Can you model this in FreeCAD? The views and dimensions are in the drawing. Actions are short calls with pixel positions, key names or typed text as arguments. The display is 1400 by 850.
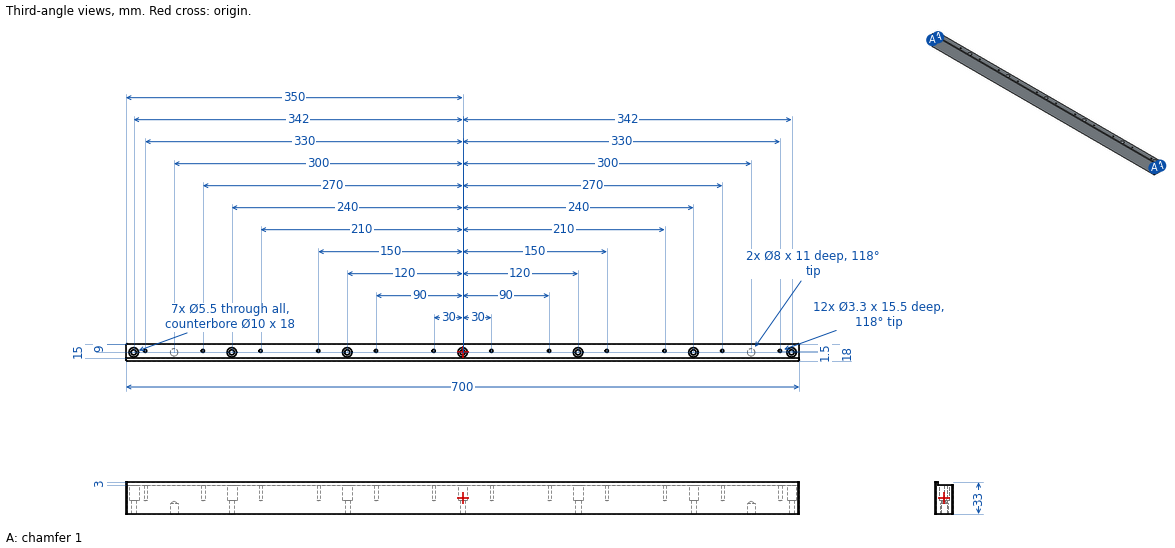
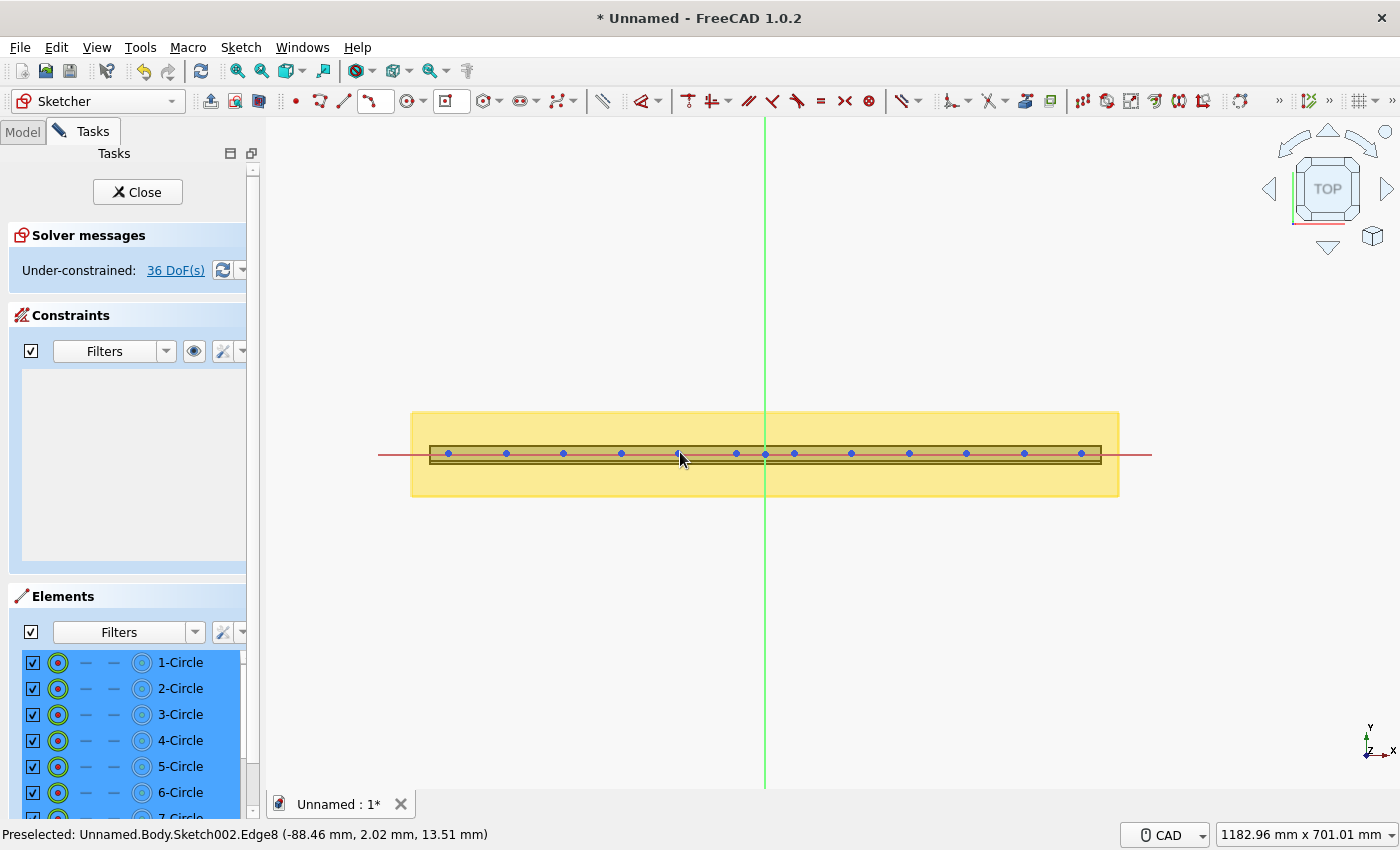
scroll(623, 452, up, 11)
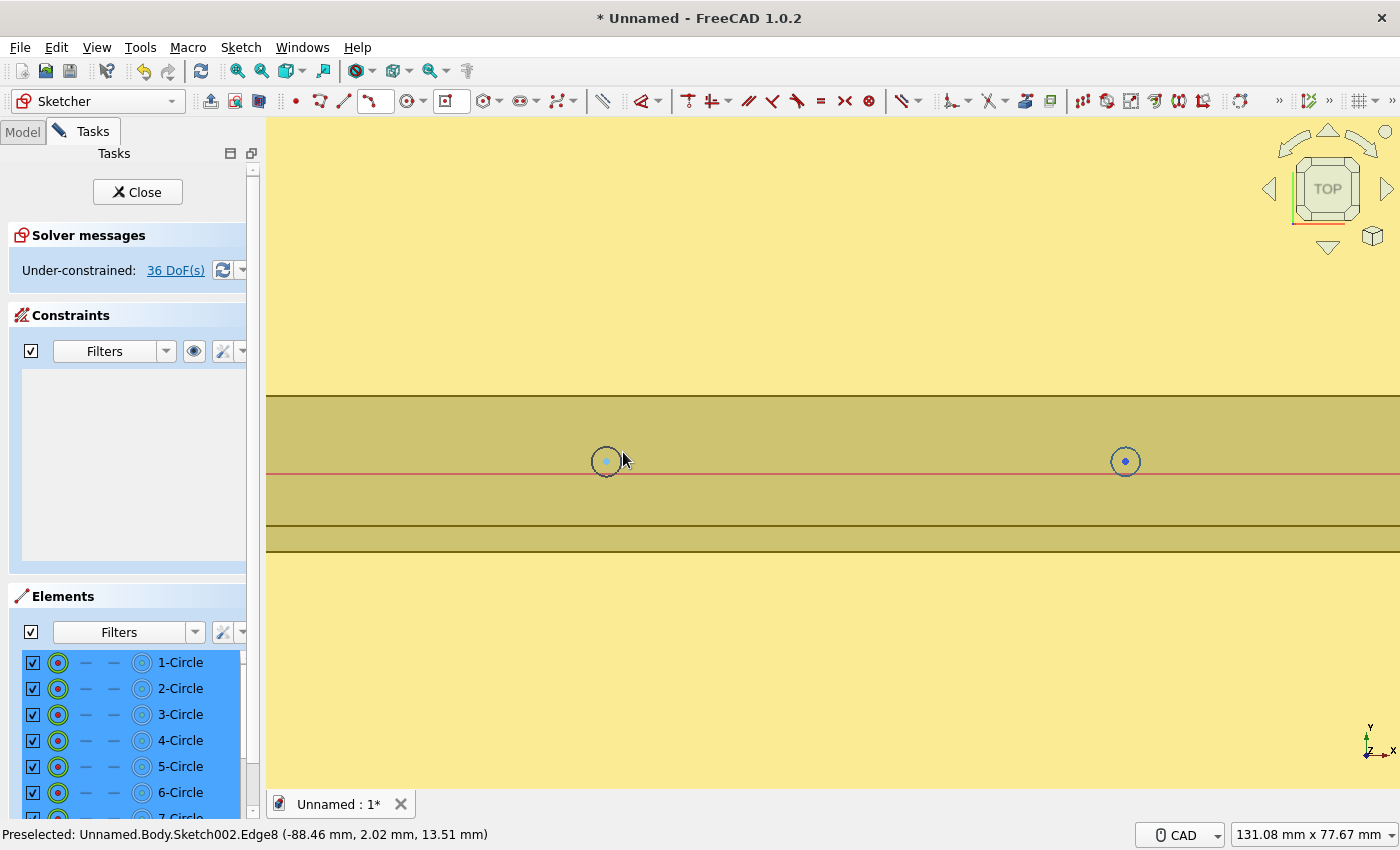
click(617, 451)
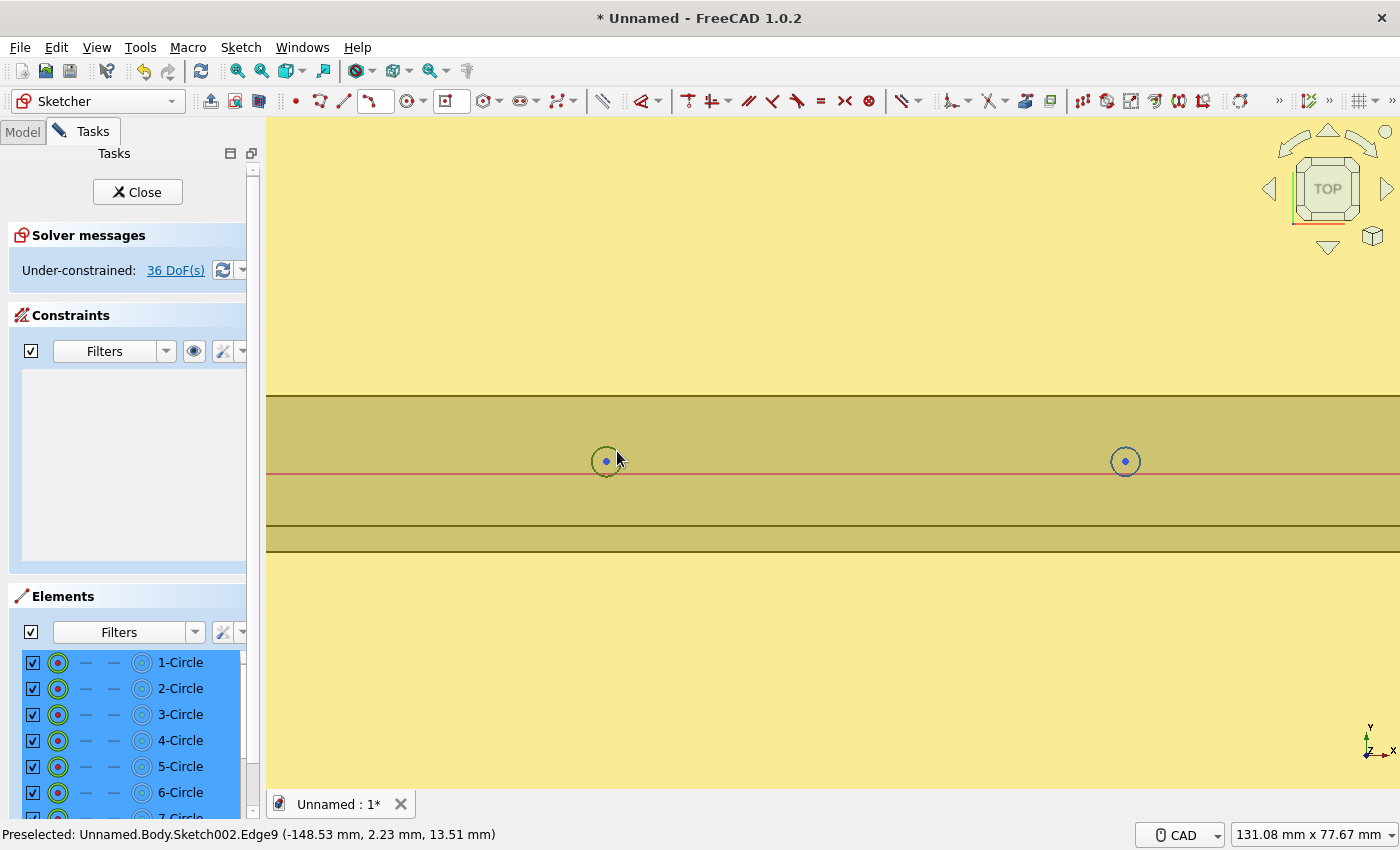
scroll(622, 452, down, 11)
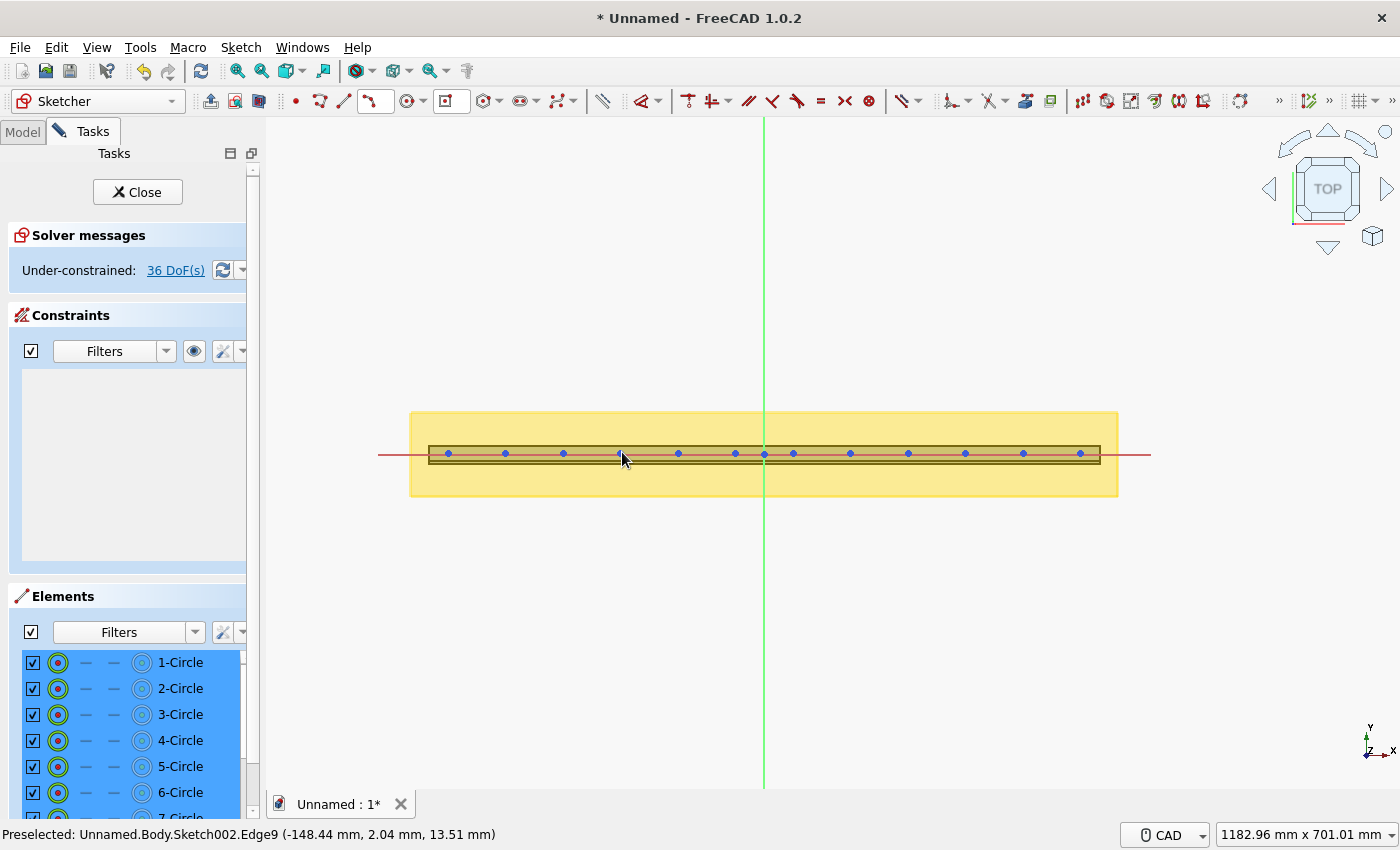
scroll(449, 452, up, 11)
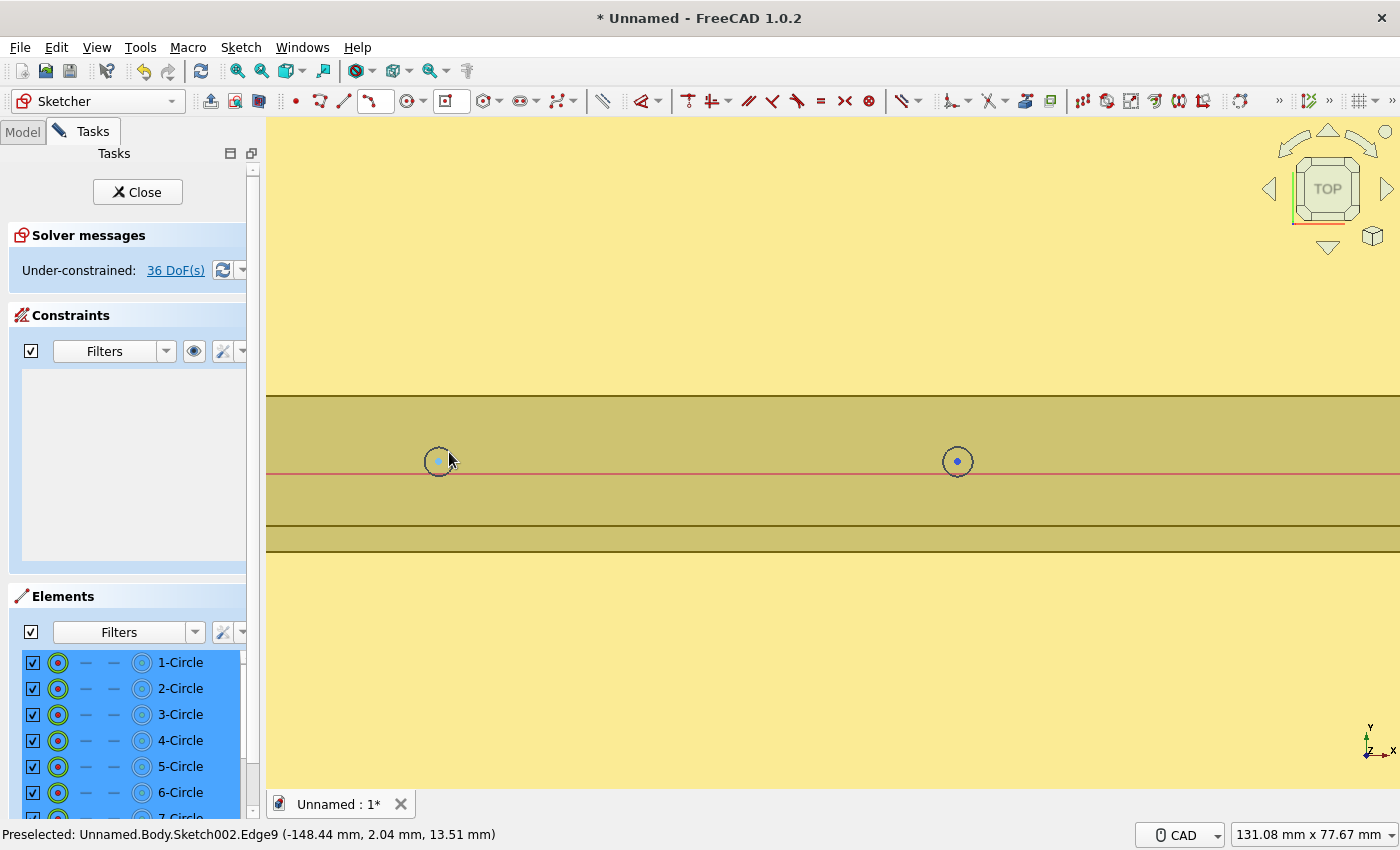
click(449, 452)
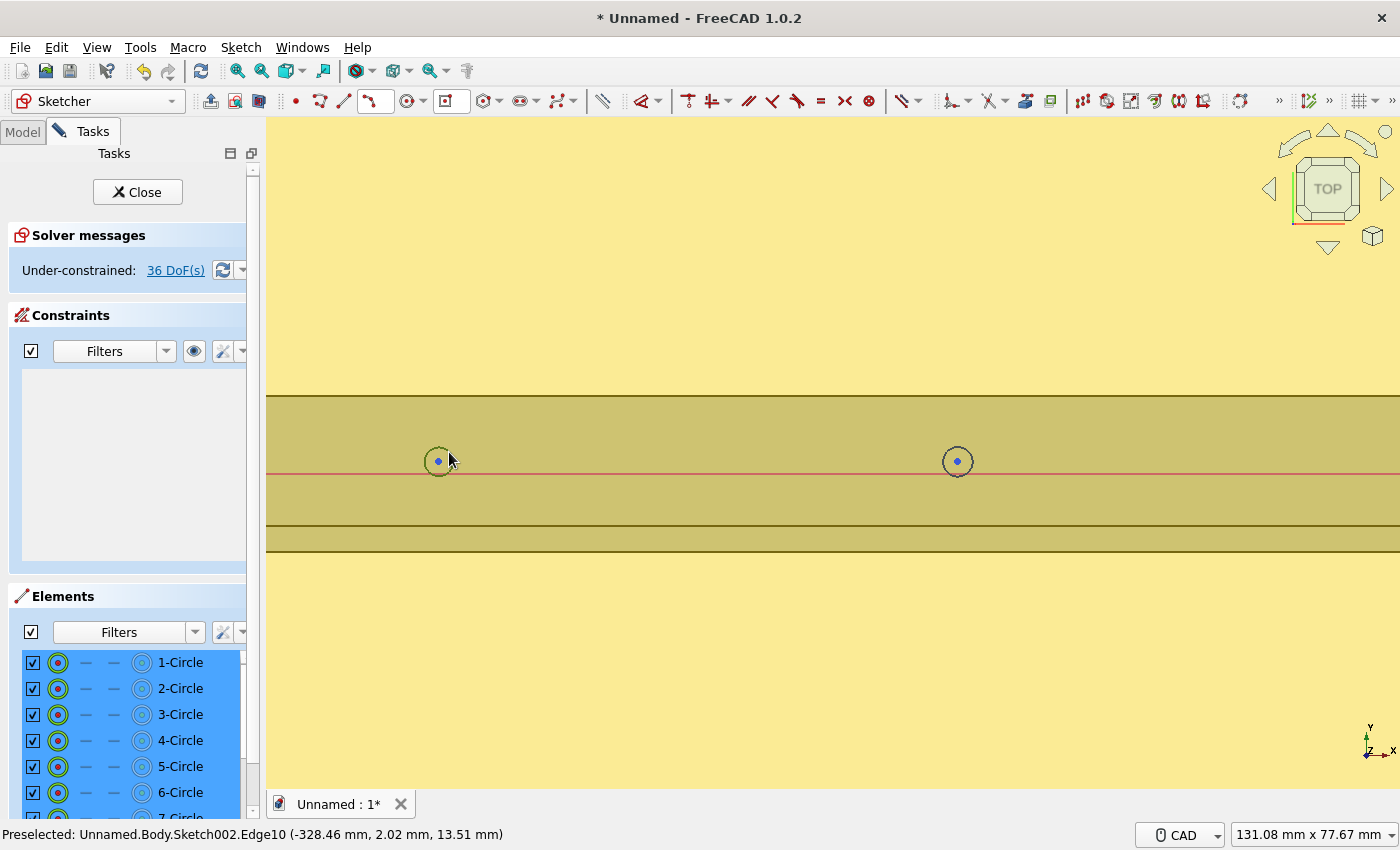
scroll(449, 452, down, 11)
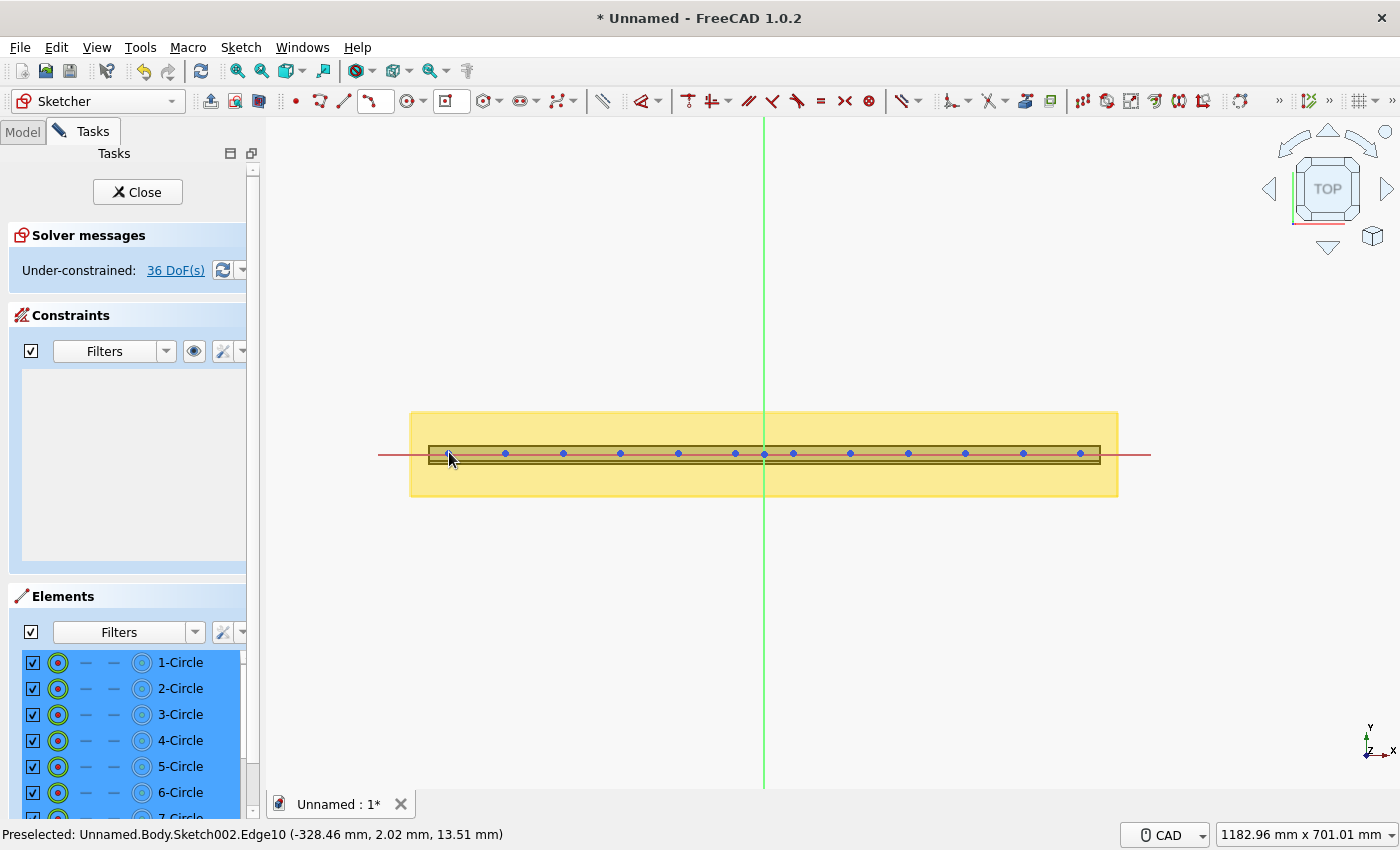
scroll(564, 452, up, 11)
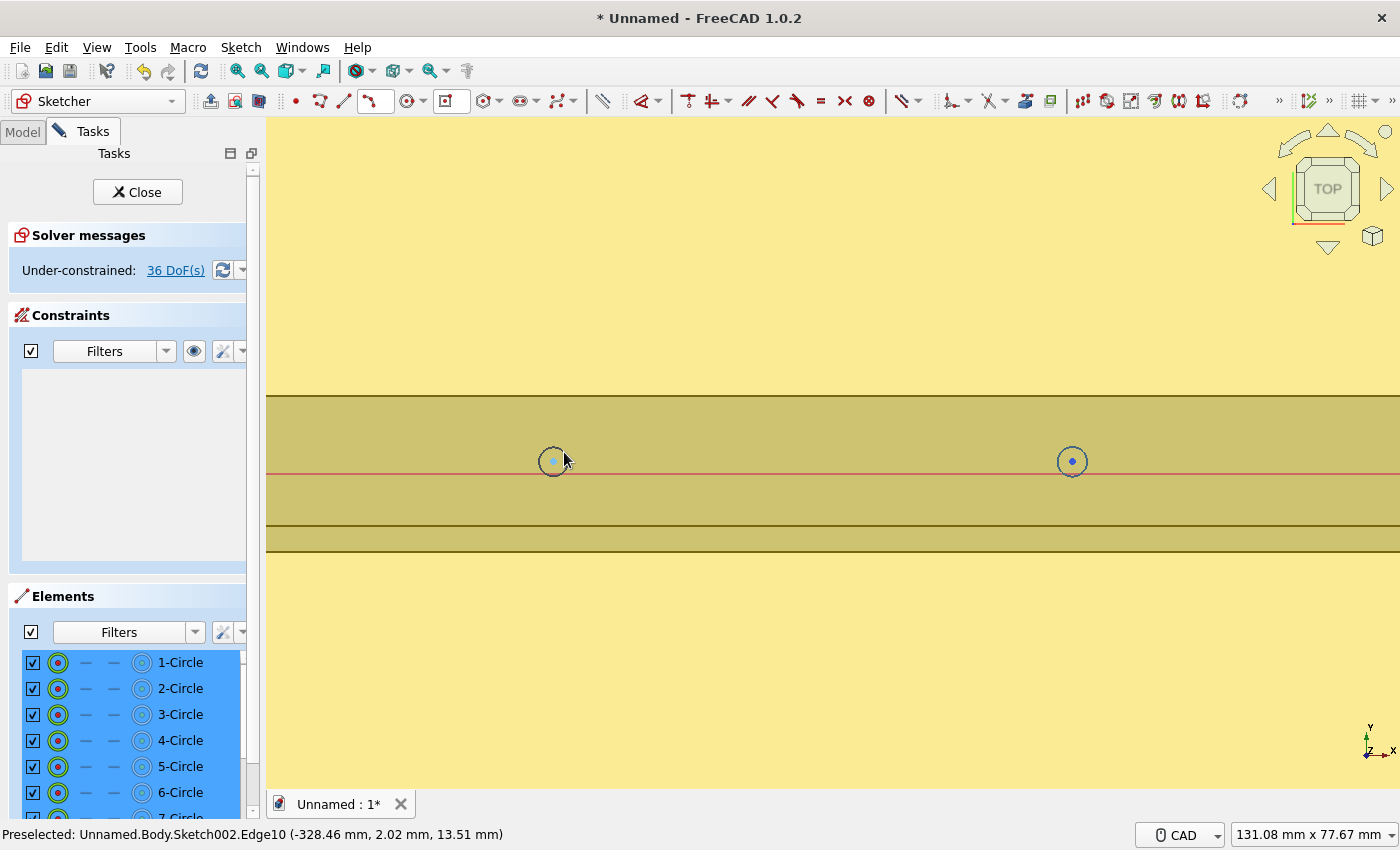
click(564, 452)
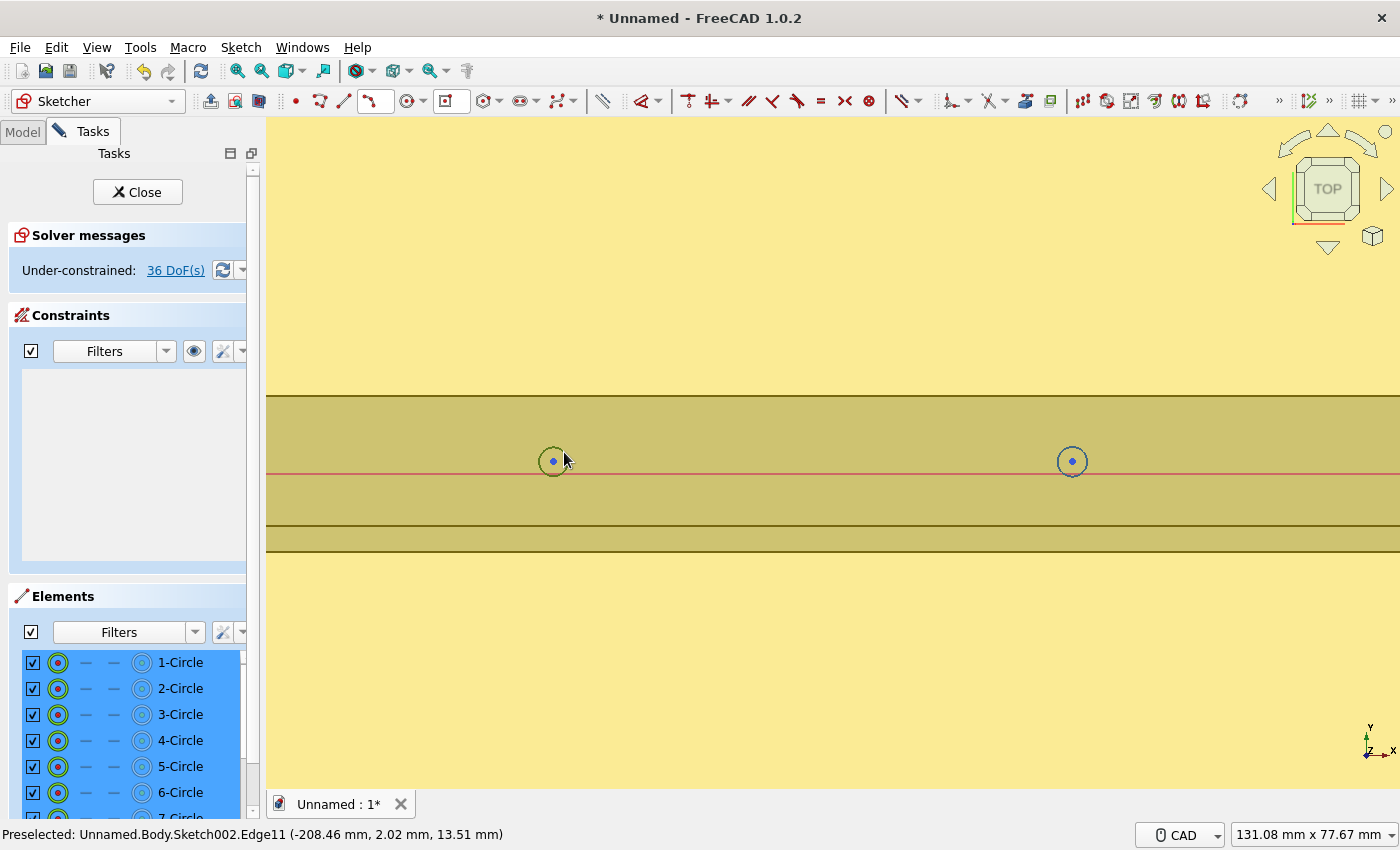
scroll(564, 452, down, 11)